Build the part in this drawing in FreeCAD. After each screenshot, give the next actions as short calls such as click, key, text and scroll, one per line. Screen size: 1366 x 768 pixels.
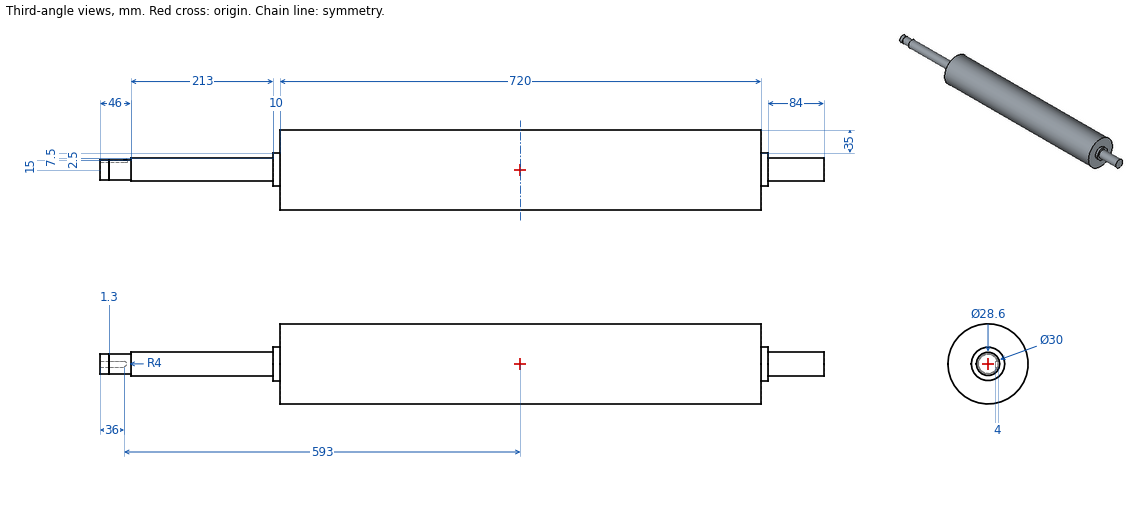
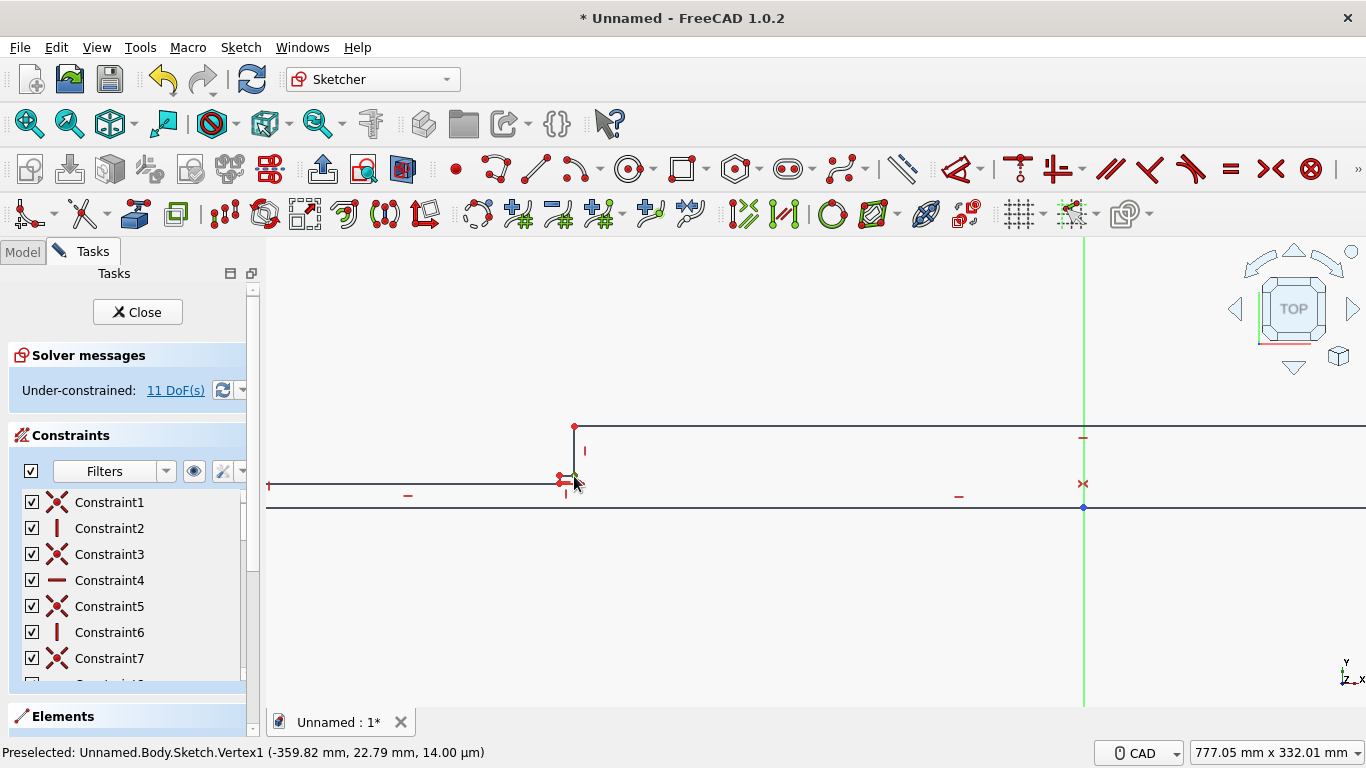
scroll(574, 477, down, 4)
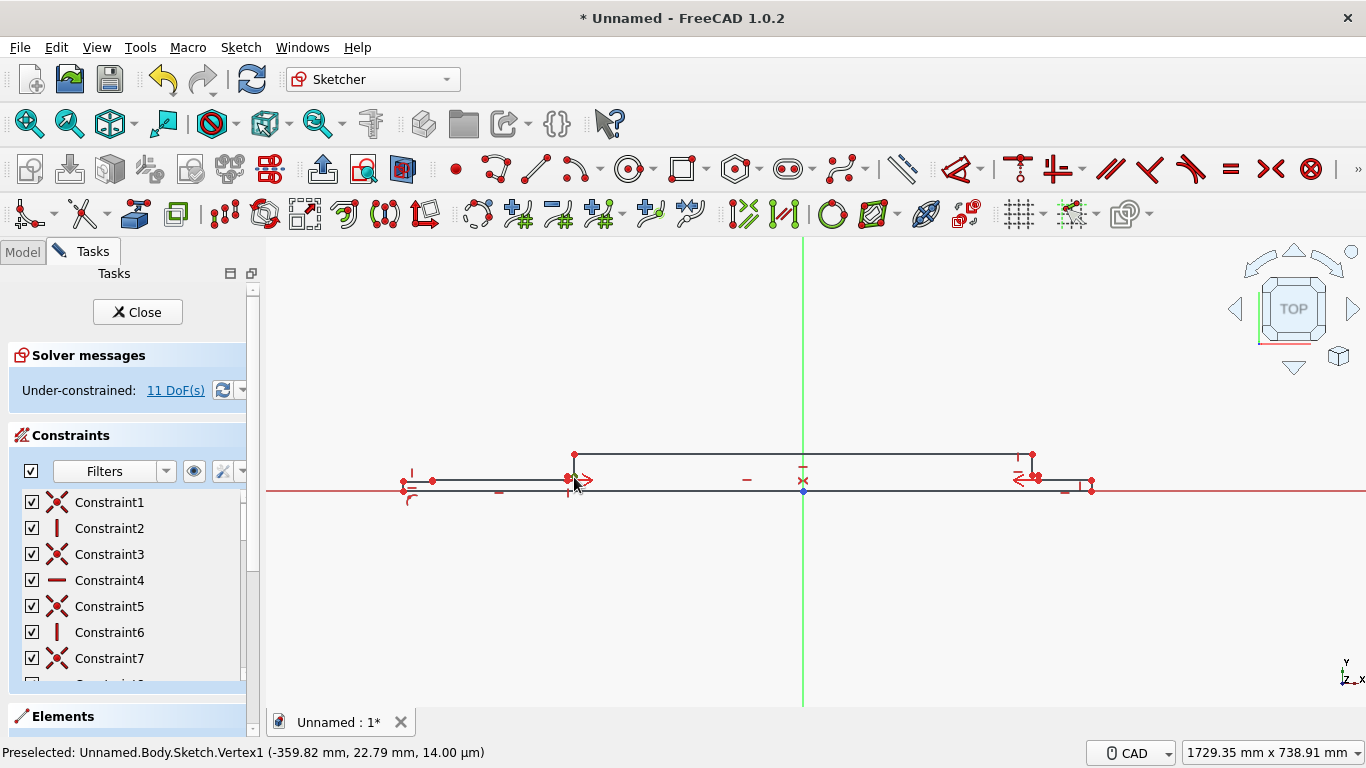
scroll(1032, 476, up, 4)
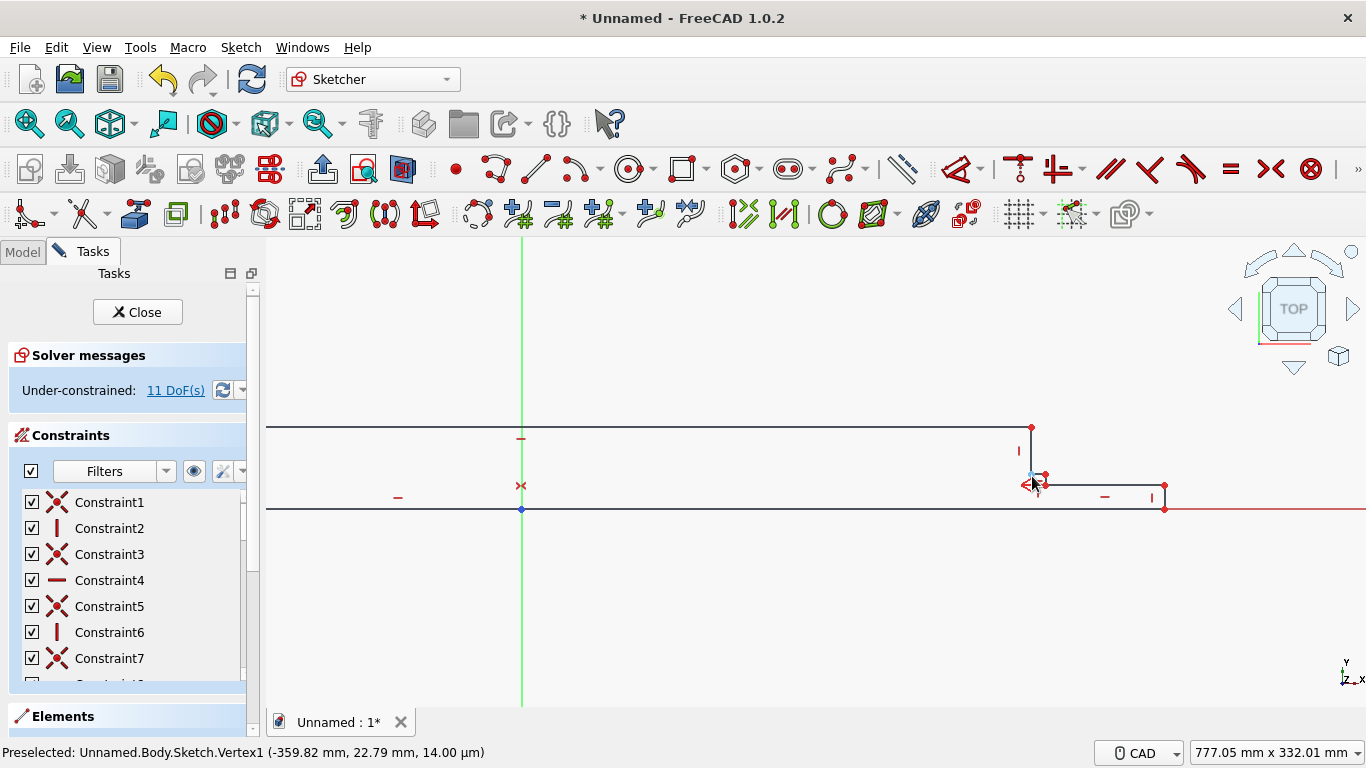
click(1031, 474)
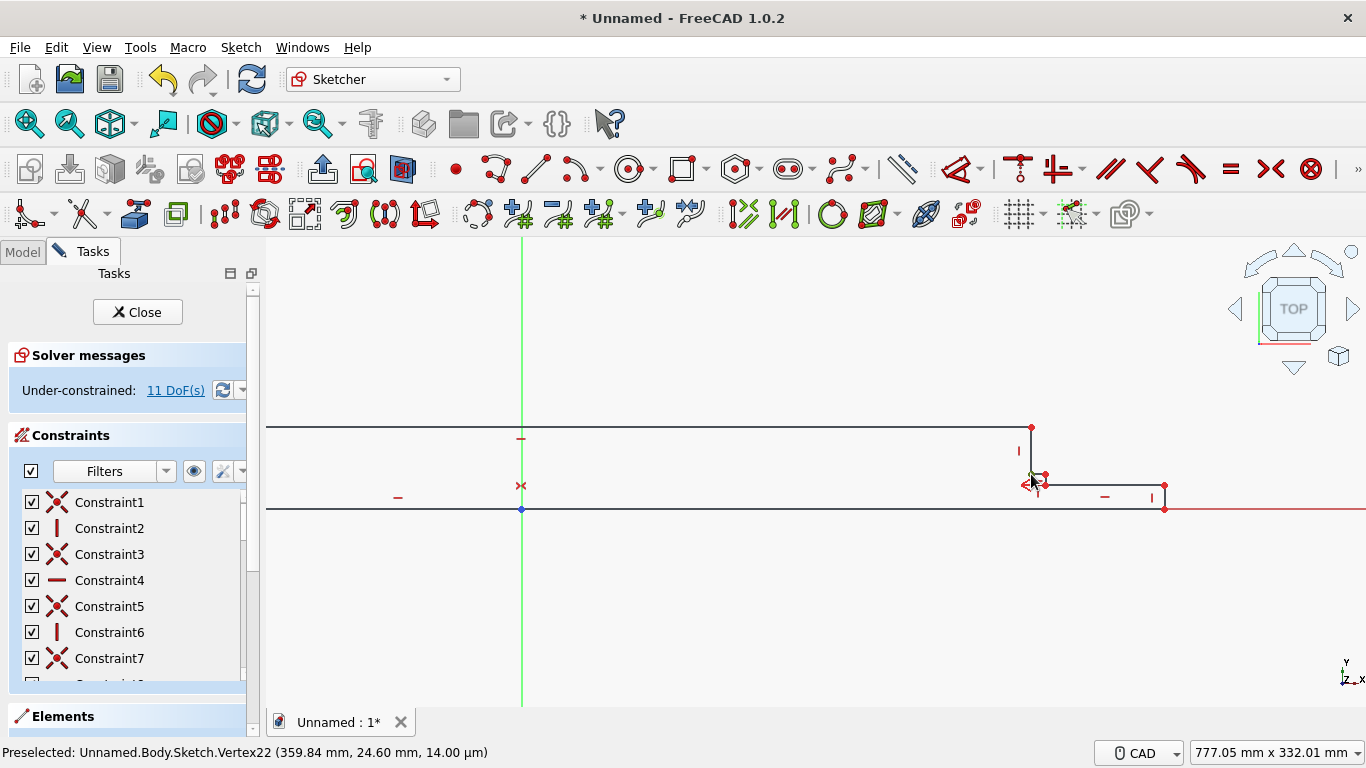
click(522, 649)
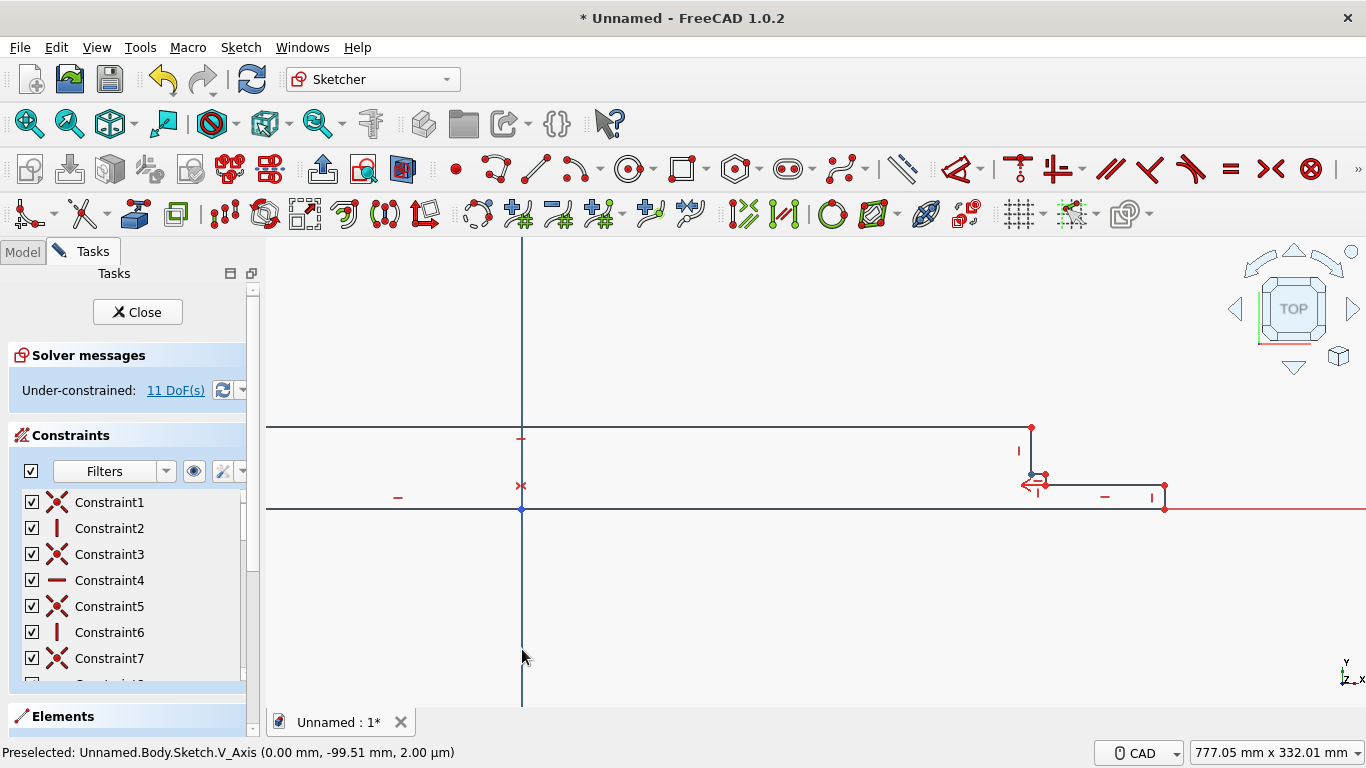
click(1272, 170)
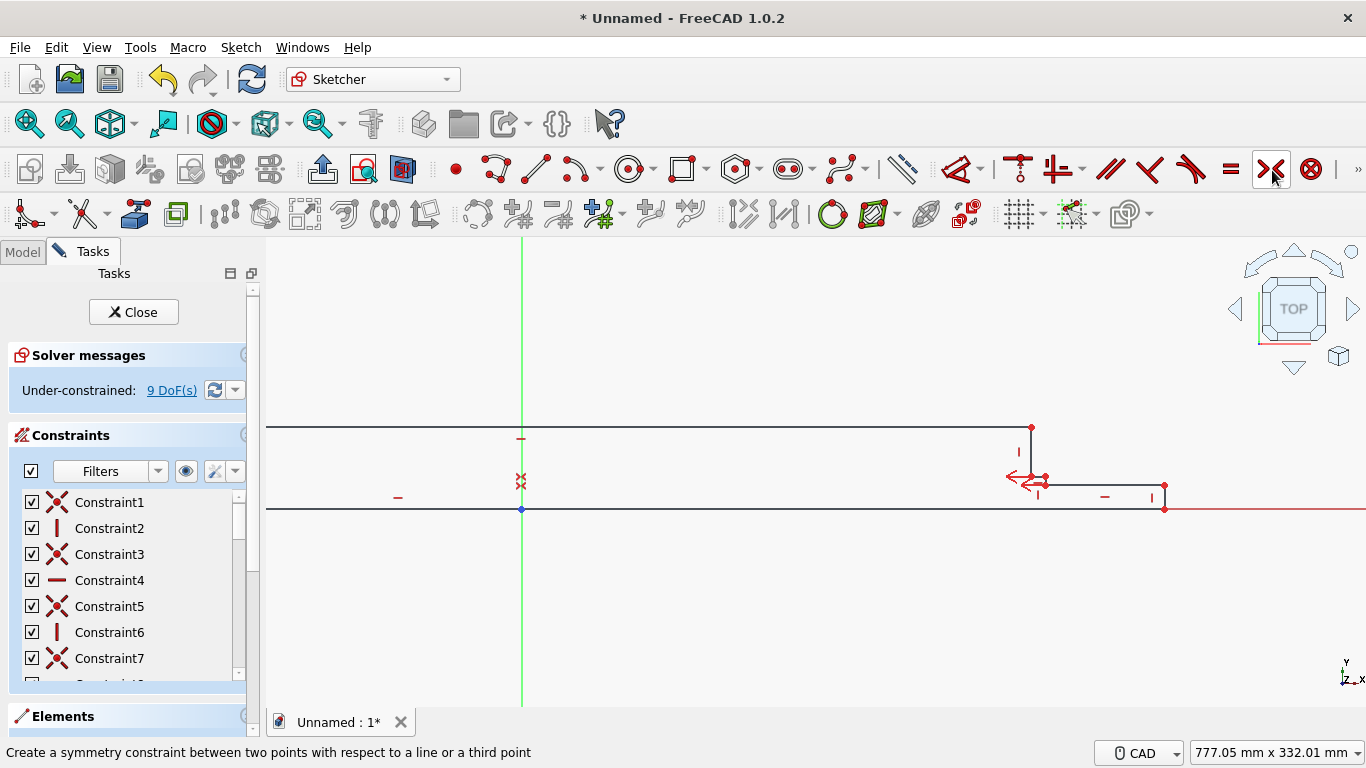
click(956, 170)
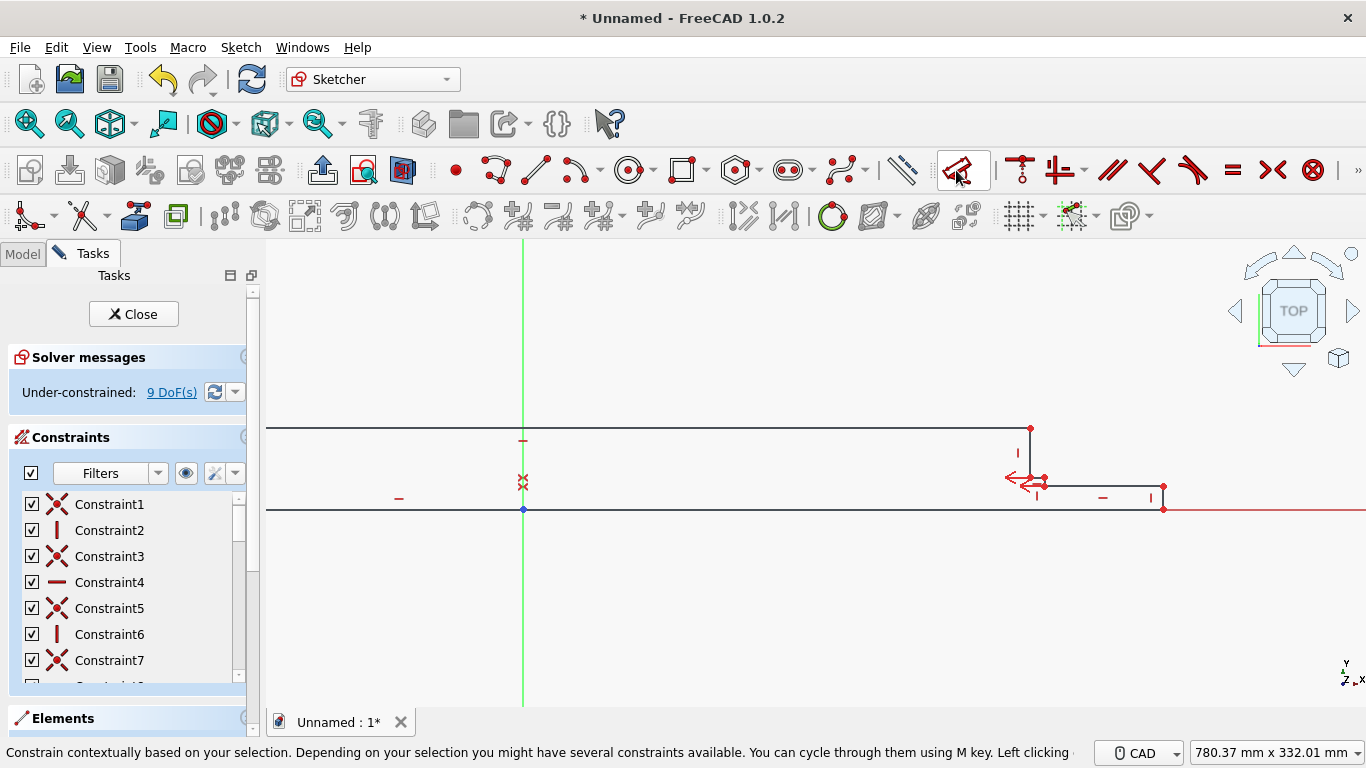
scroll(1031, 477, down, 4)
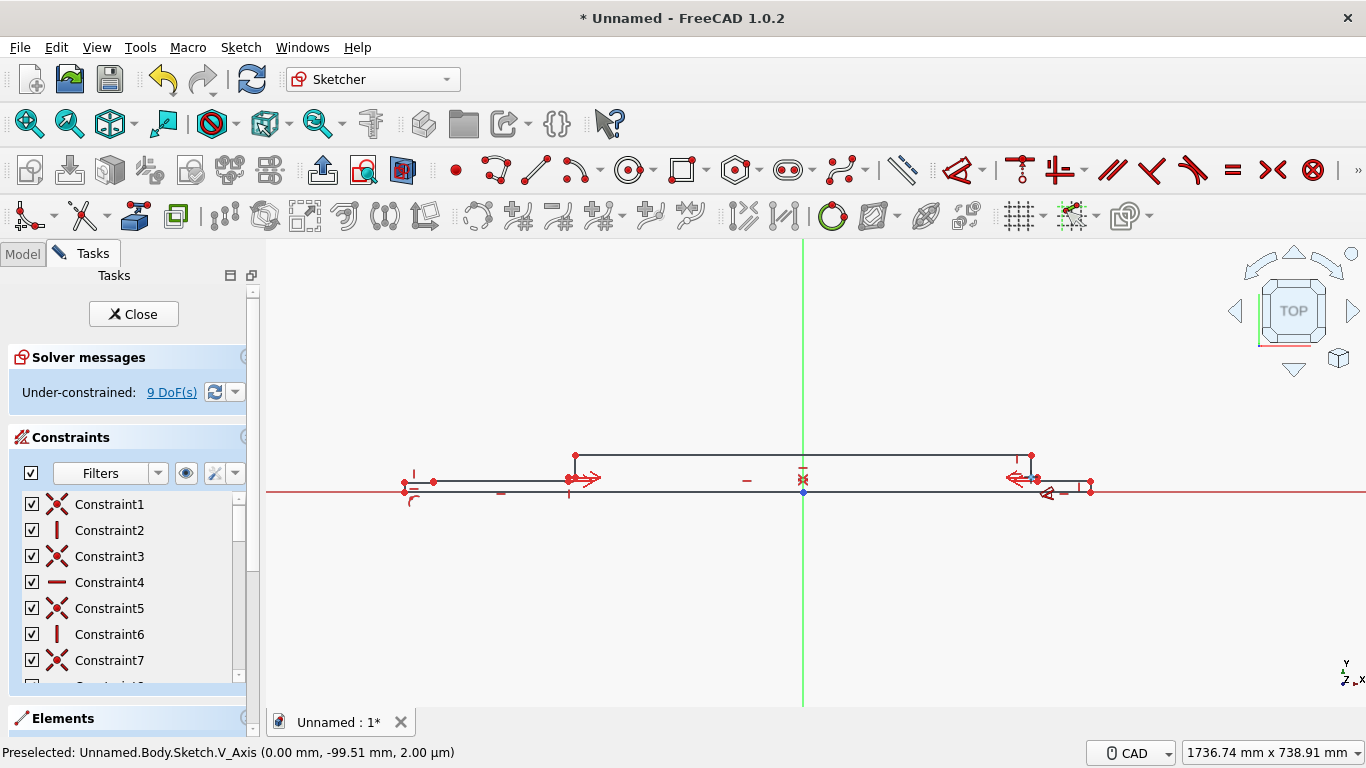
scroll(572, 478, up, 10)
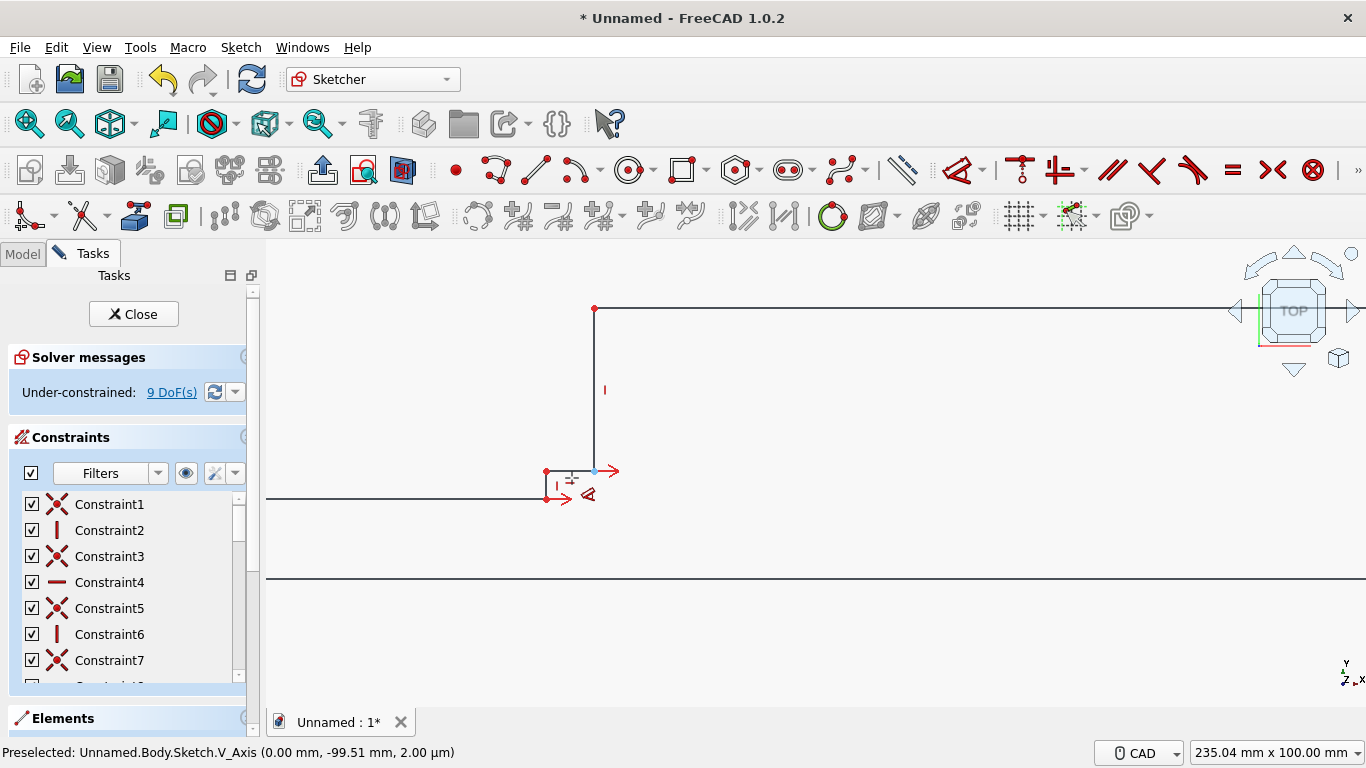
click(570, 471)
click(570, 505)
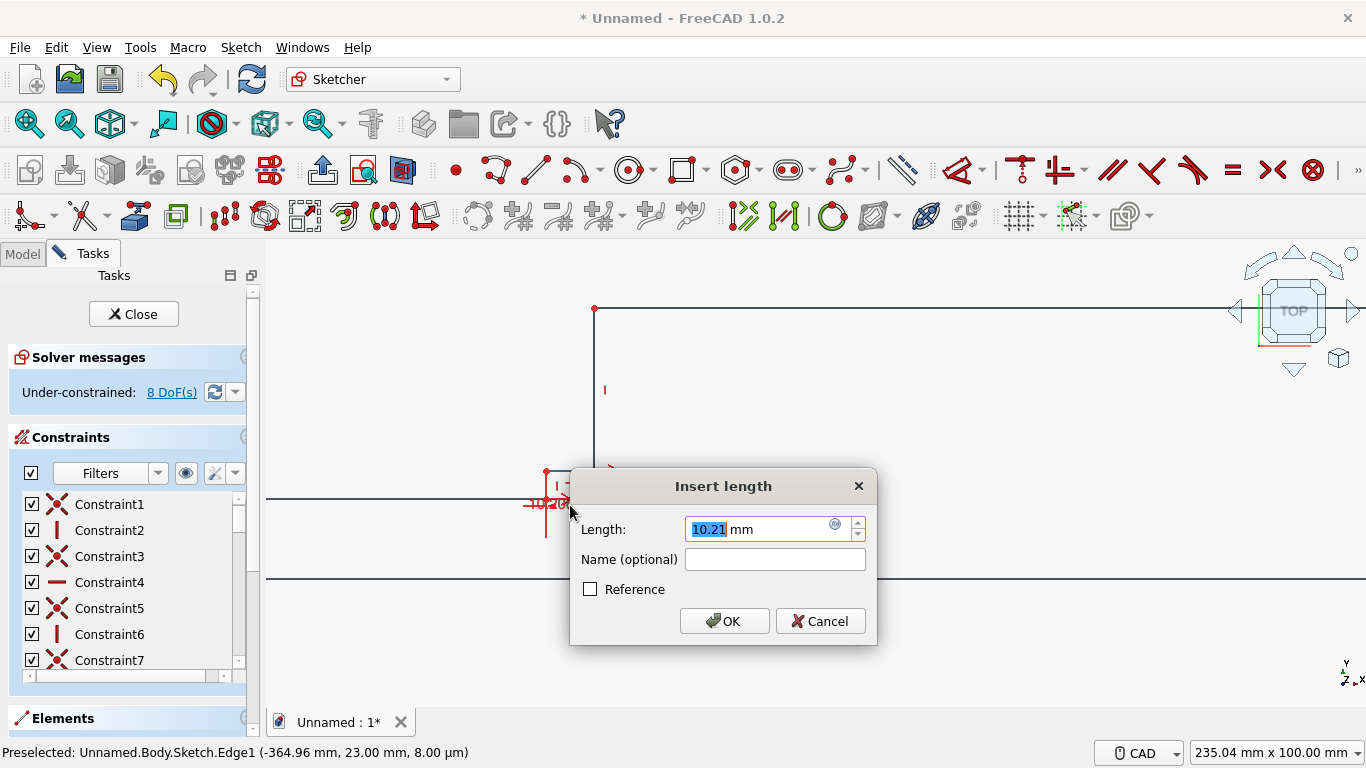
text(10)
key(Return)